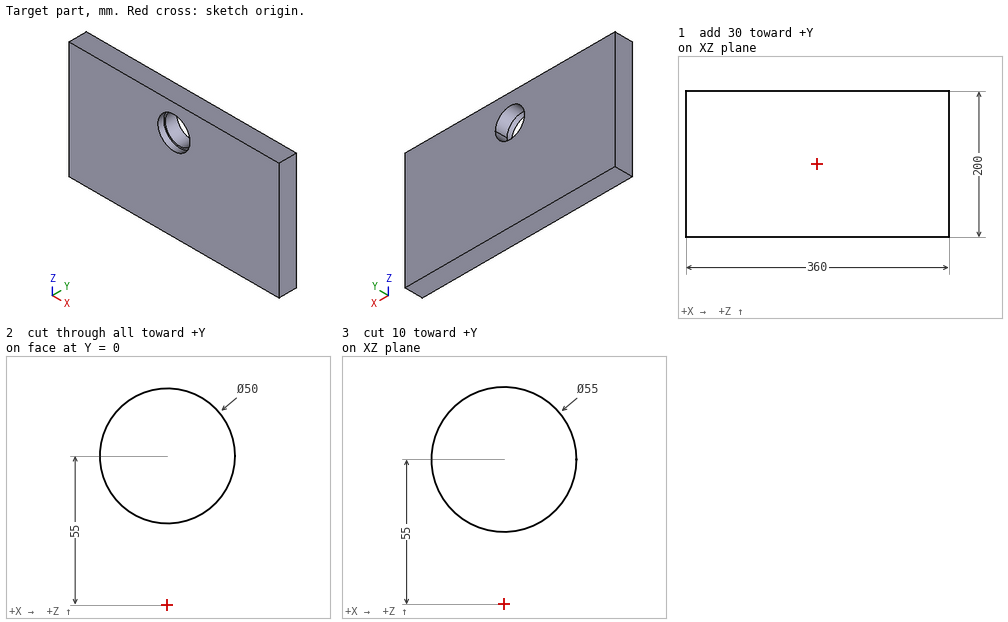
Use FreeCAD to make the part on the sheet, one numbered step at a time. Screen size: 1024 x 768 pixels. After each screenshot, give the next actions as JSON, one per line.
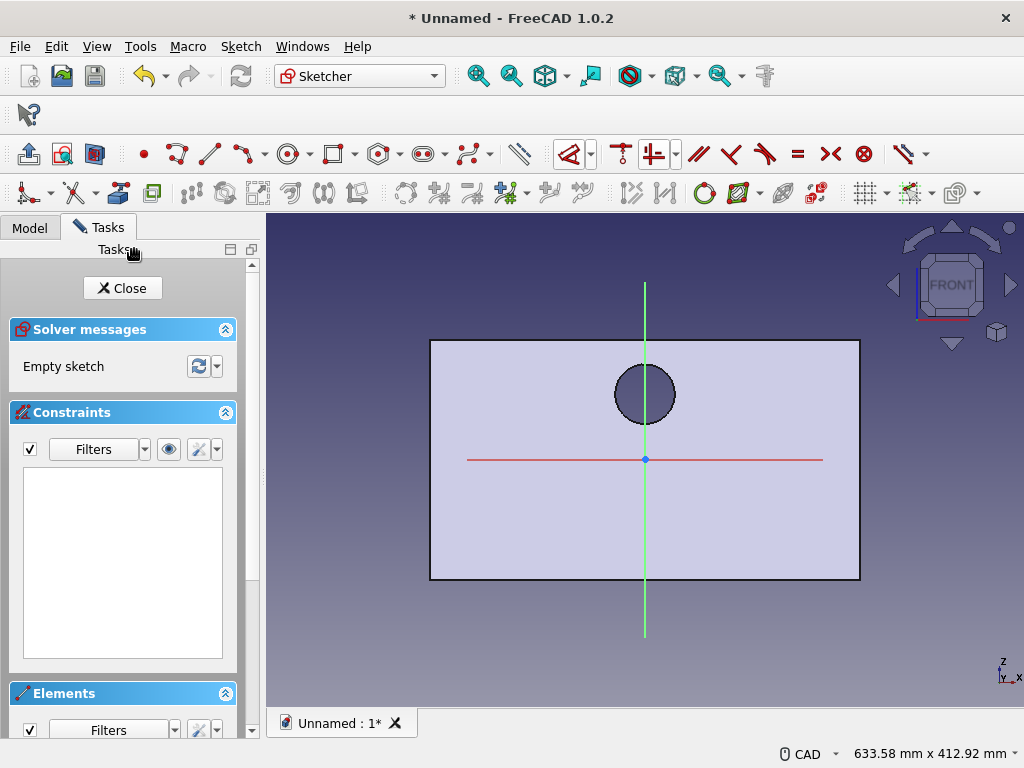
{"action": "scroll", "coordinate": [675, 389], "scroll_direction": "up", "scroll_amount": 6}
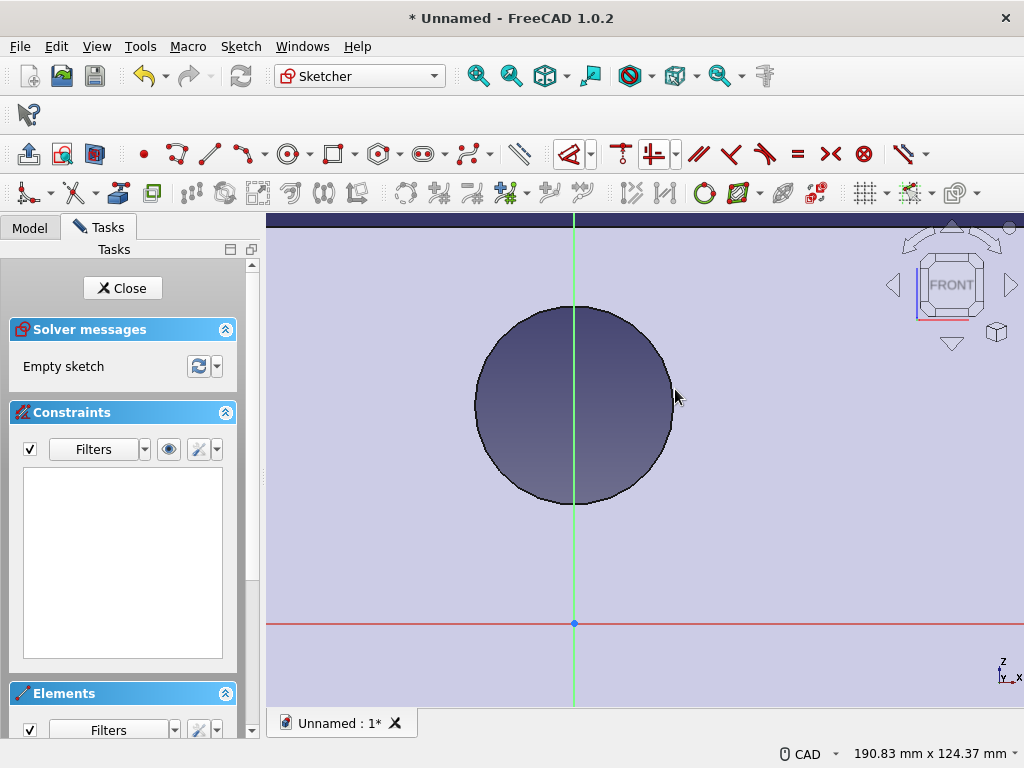
{"action": "key", "text": "g c"}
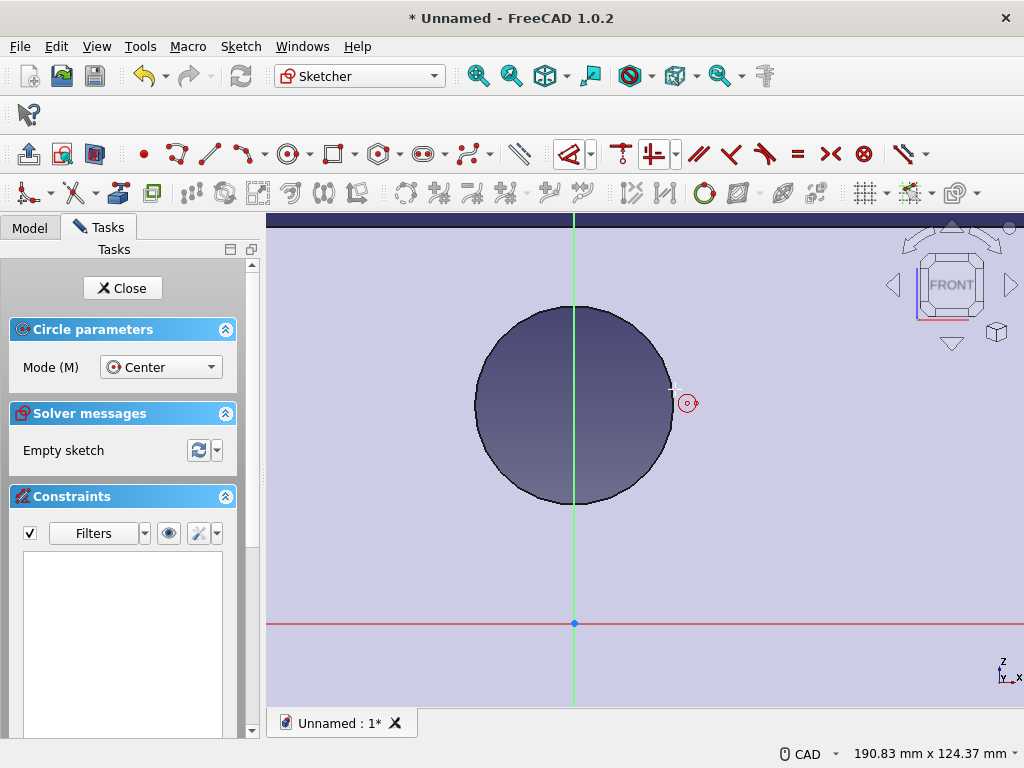
{"action": "left_click", "coordinate": [574, 405]}
{"action": "left_click", "coordinate": [651, 328]}
{"action": "key", "text": "Escape"}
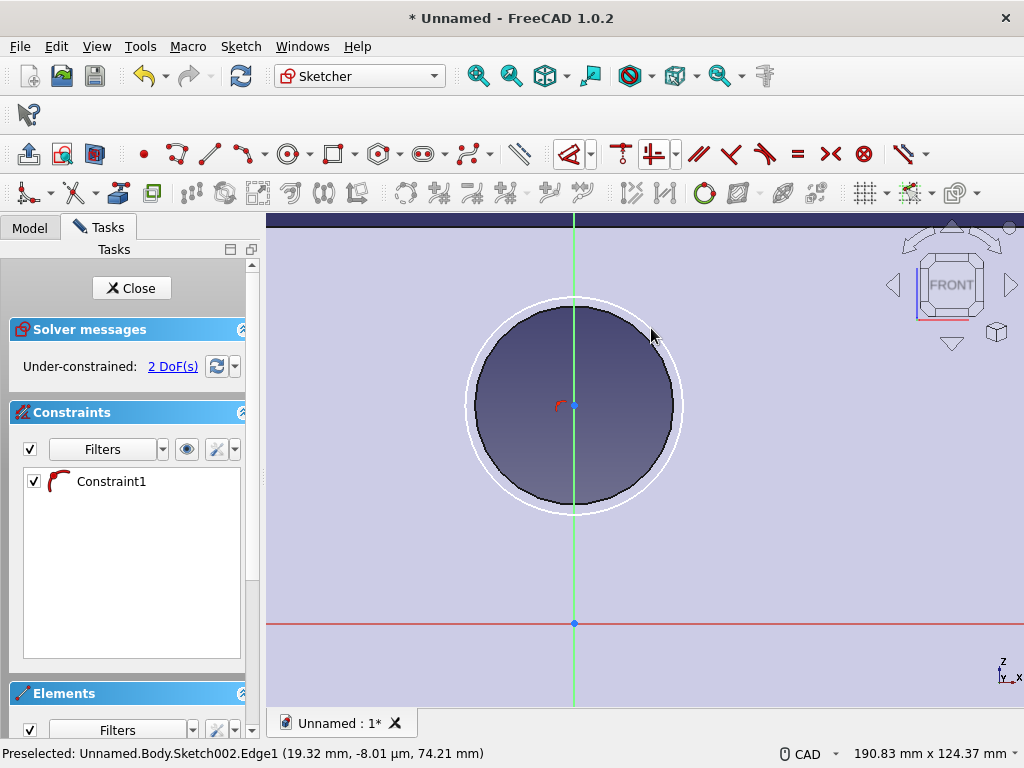
{"action": "left_click", "coordinate": [651, 329]}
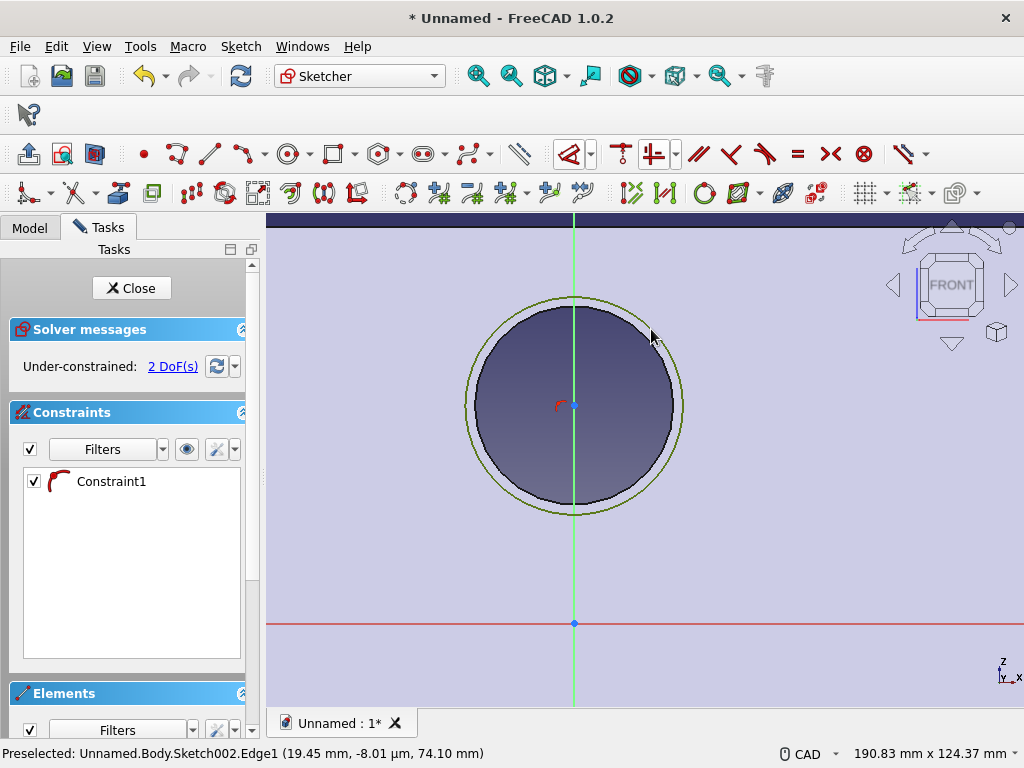
{"action": "key", "text": "k o"}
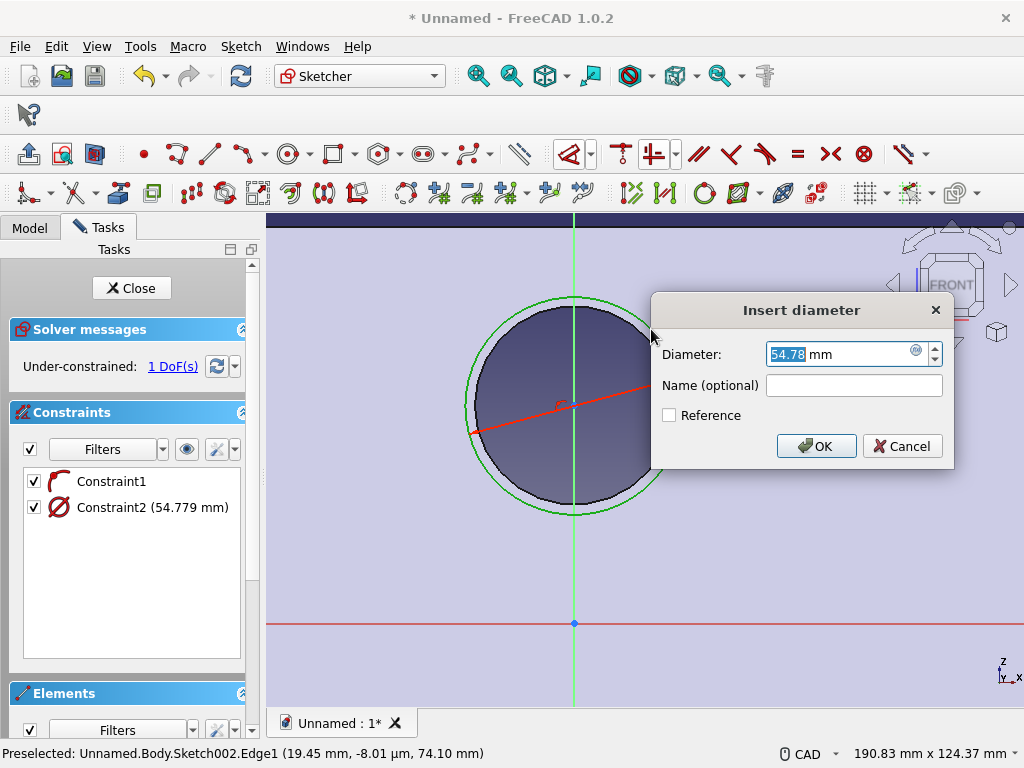
{"action": "type", "text": "55"}
{"action": "key", "text": "Return"}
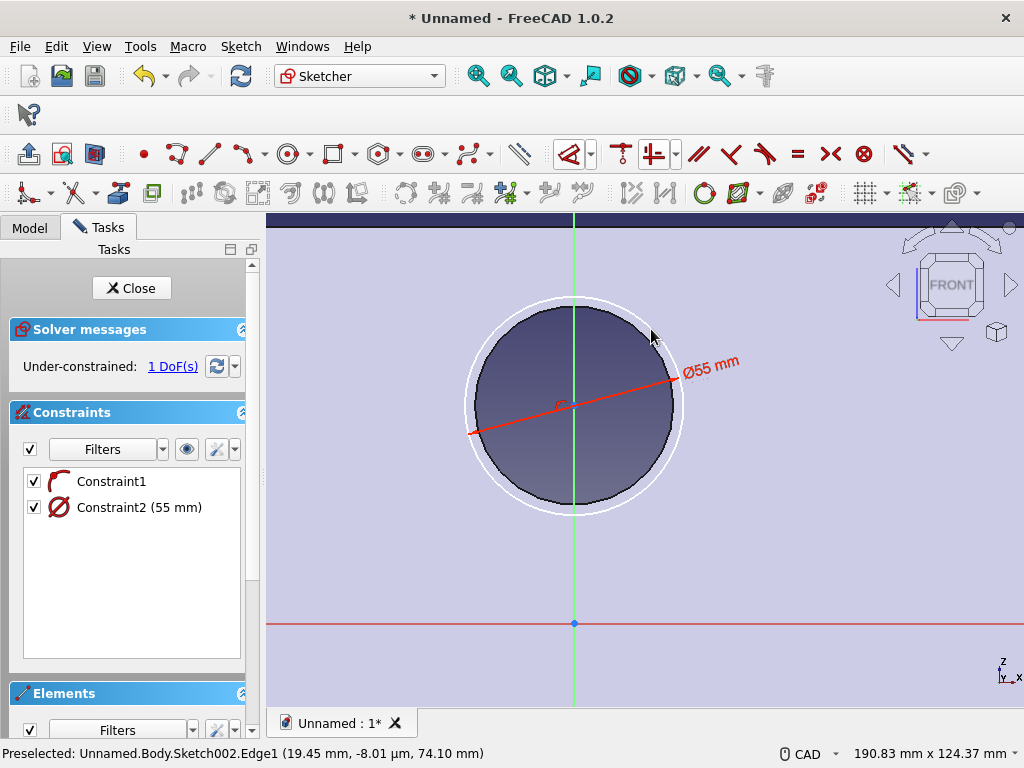
{"action": "left_click", "coordinate": [574, 406]}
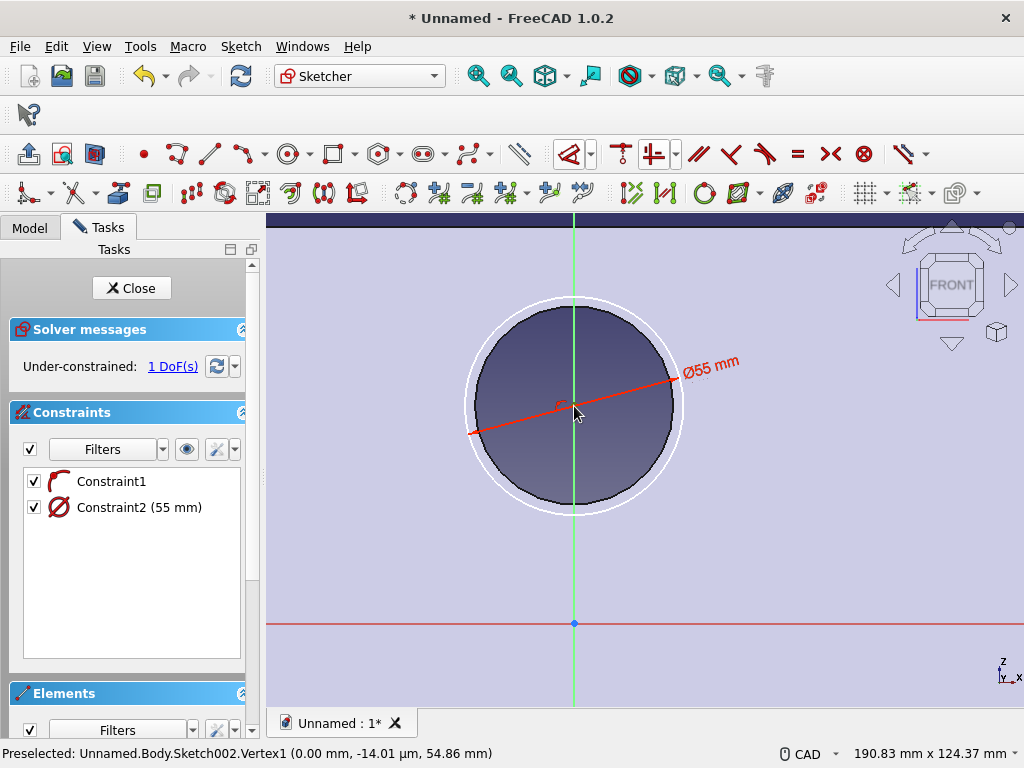
{"action": "key", "text": "i"}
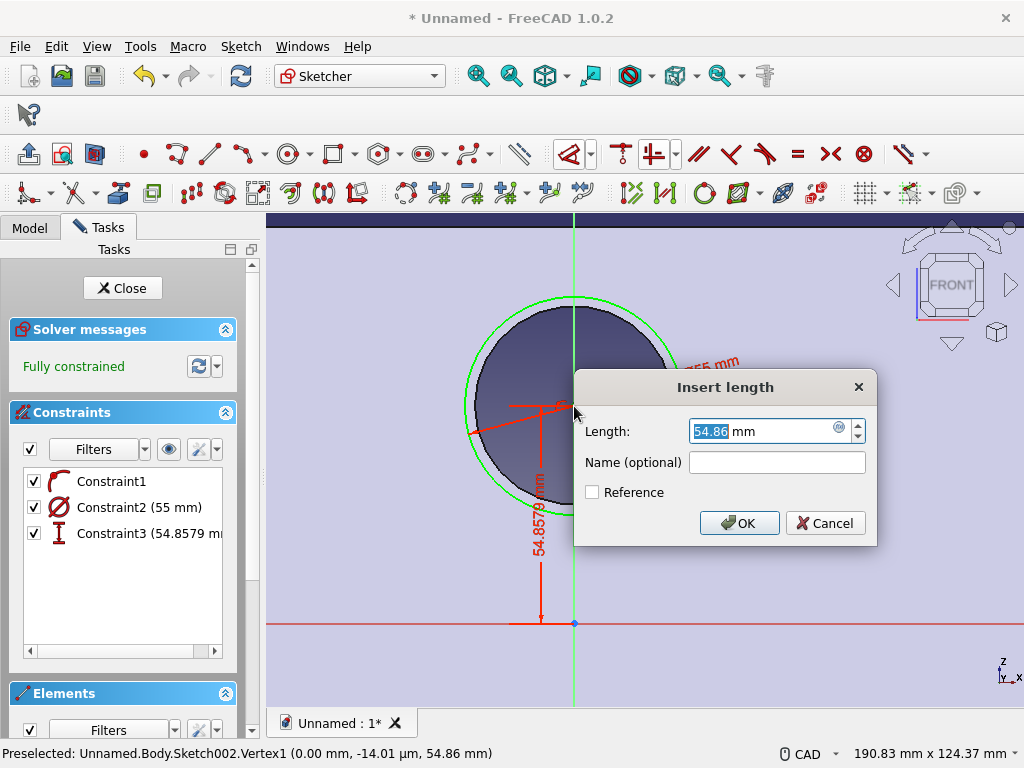
{"action": "type", "text": "55"}
{"action": "key", "text": "Return"}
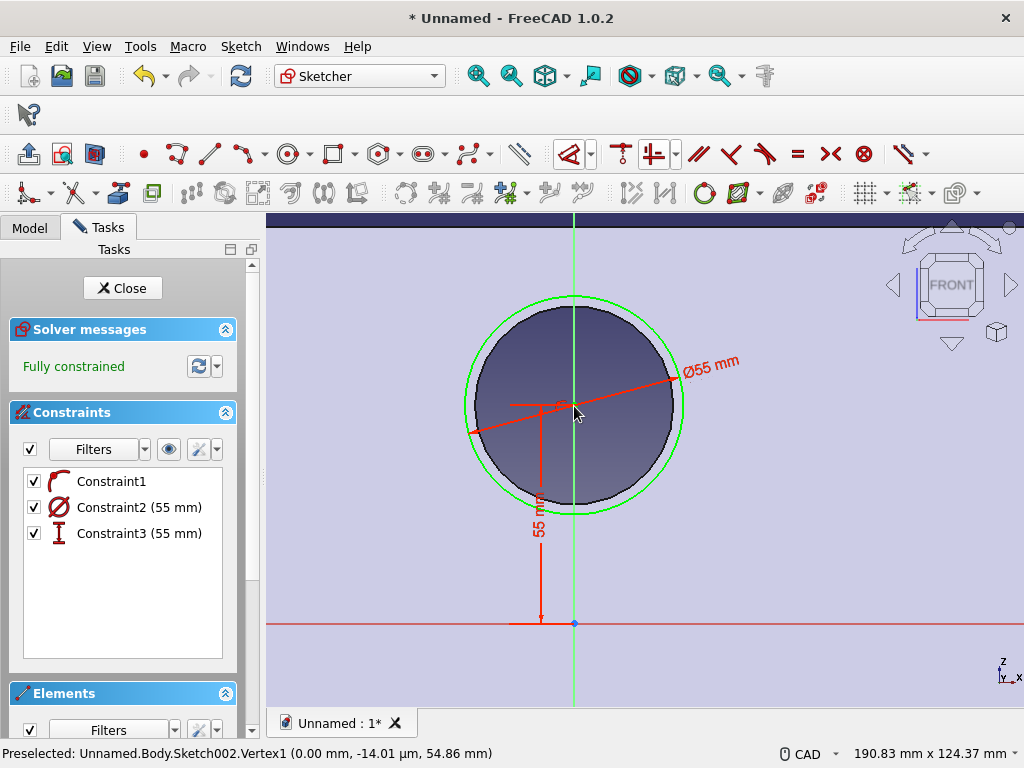
{"action": "left_click", "coordinate": [123, 288]}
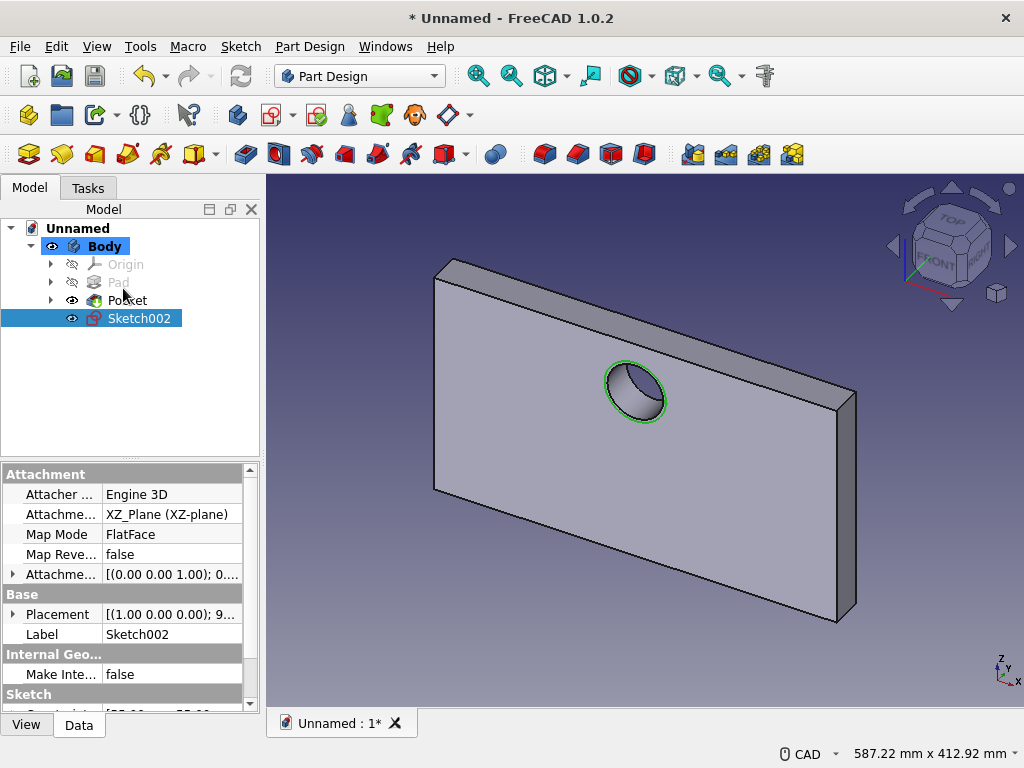
{"action": "left_click", "coordinate": [246, 154]}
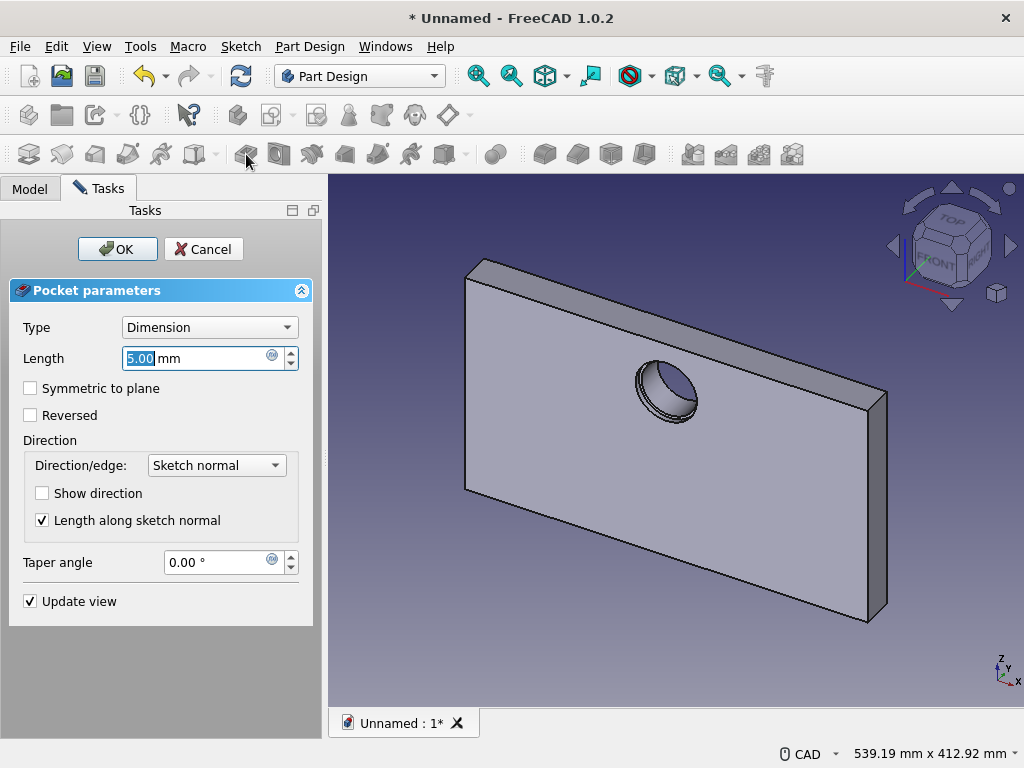
{"action": "type", "text": "10"}
{"action": "key", "text": "Tab"}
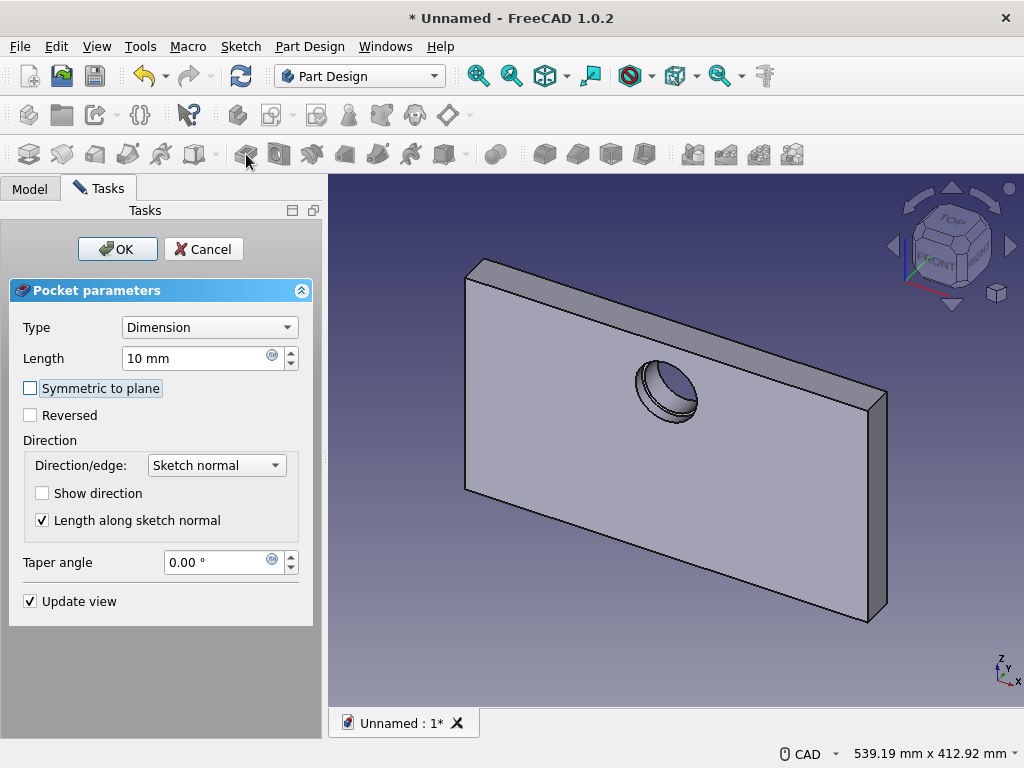
{"action": "left_click", "coordinate": [118, 249]}